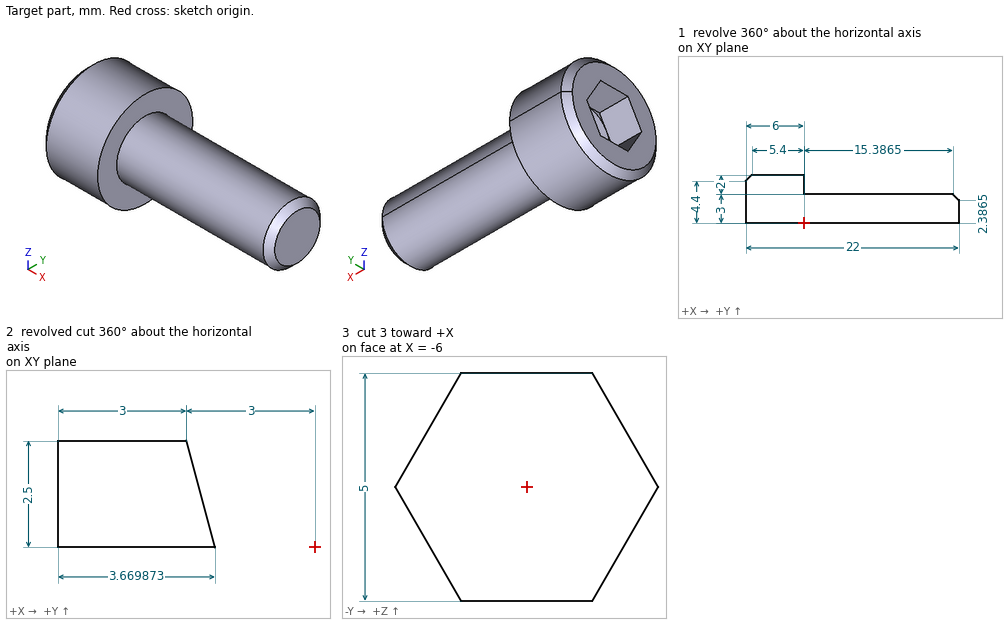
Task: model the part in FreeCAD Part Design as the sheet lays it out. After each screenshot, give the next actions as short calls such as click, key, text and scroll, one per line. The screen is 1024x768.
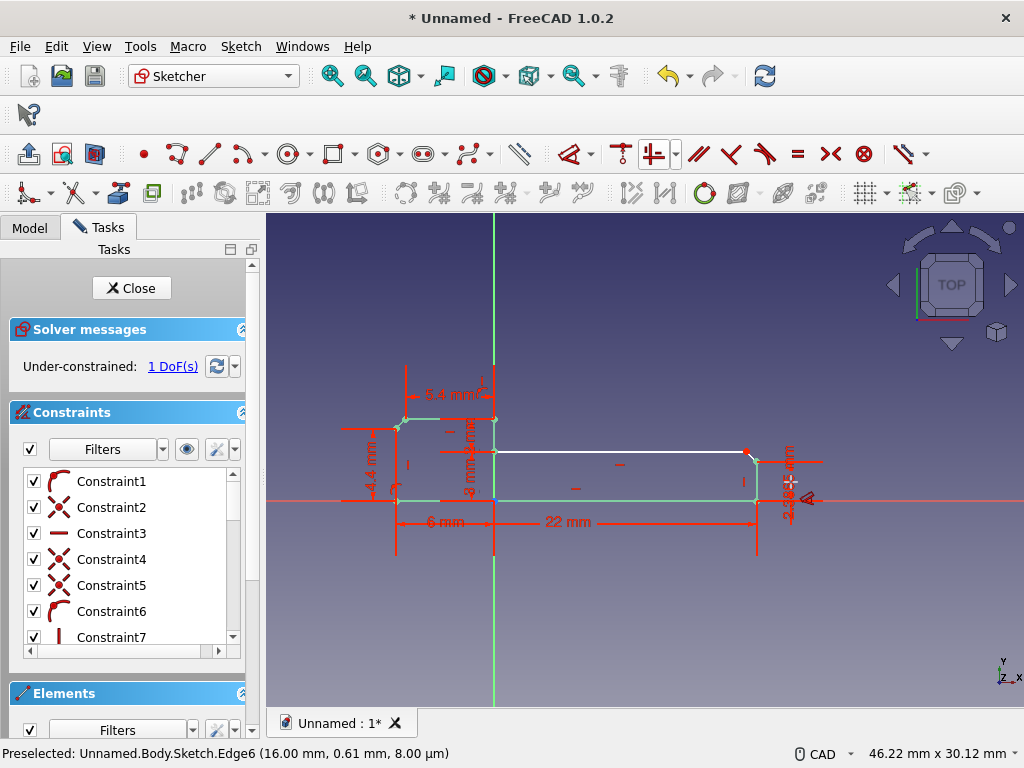
click(671, 452)
click(621, 418)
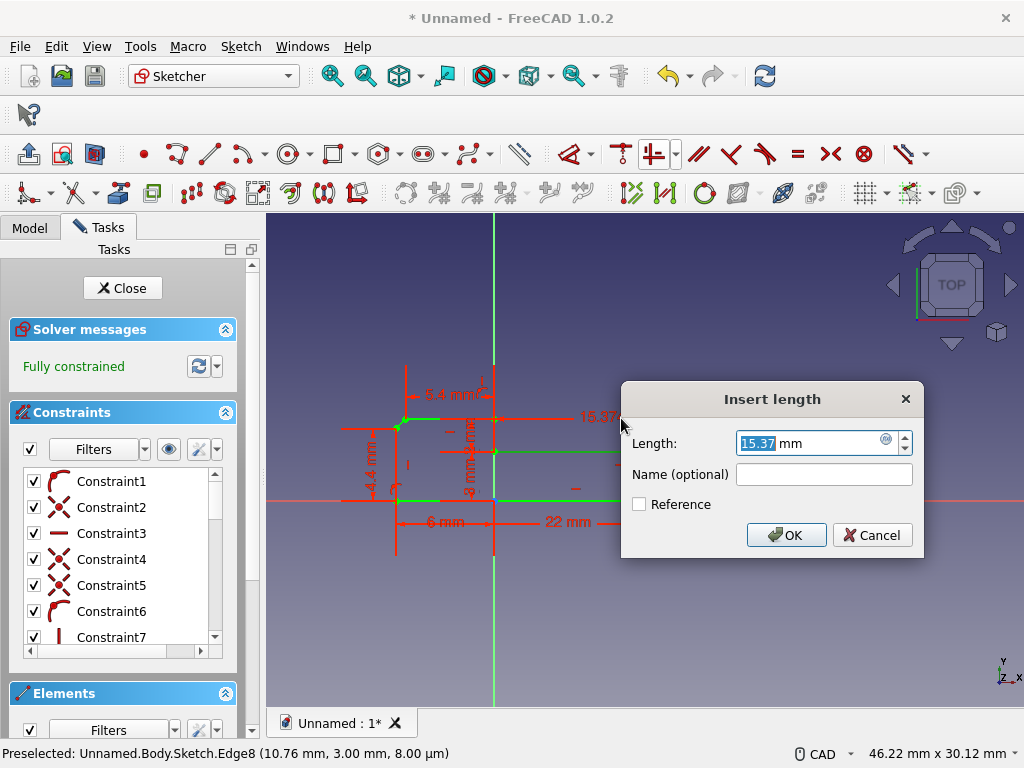
text(15.3865)
key(Return)
key(Escape)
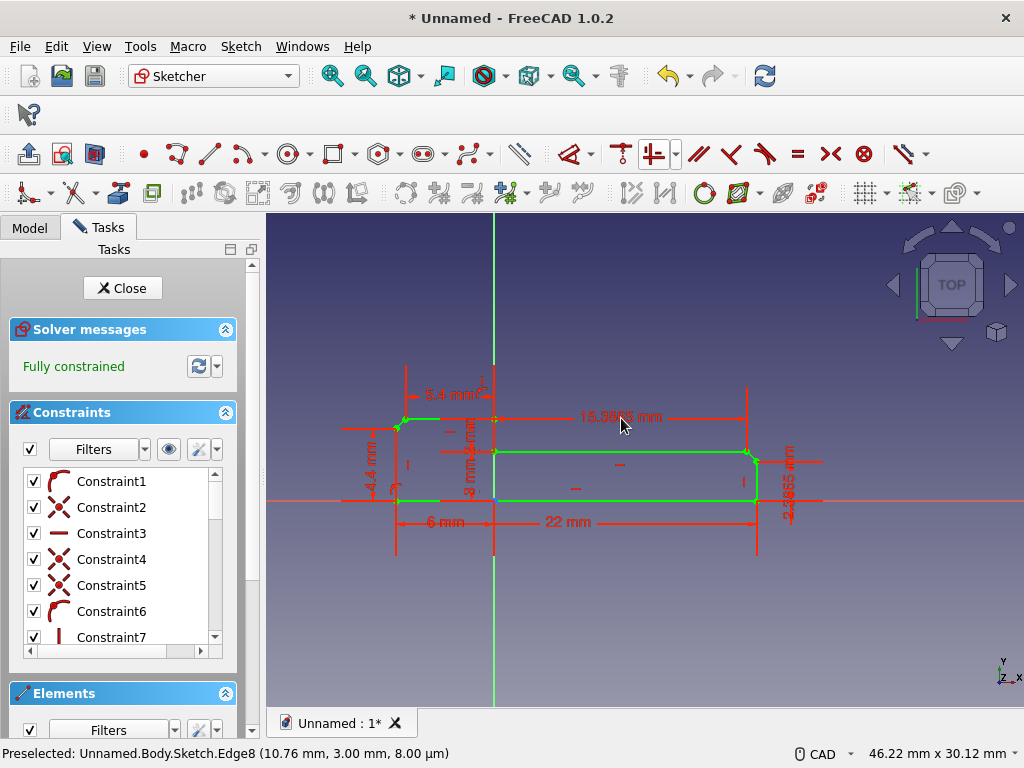
click(123, 288)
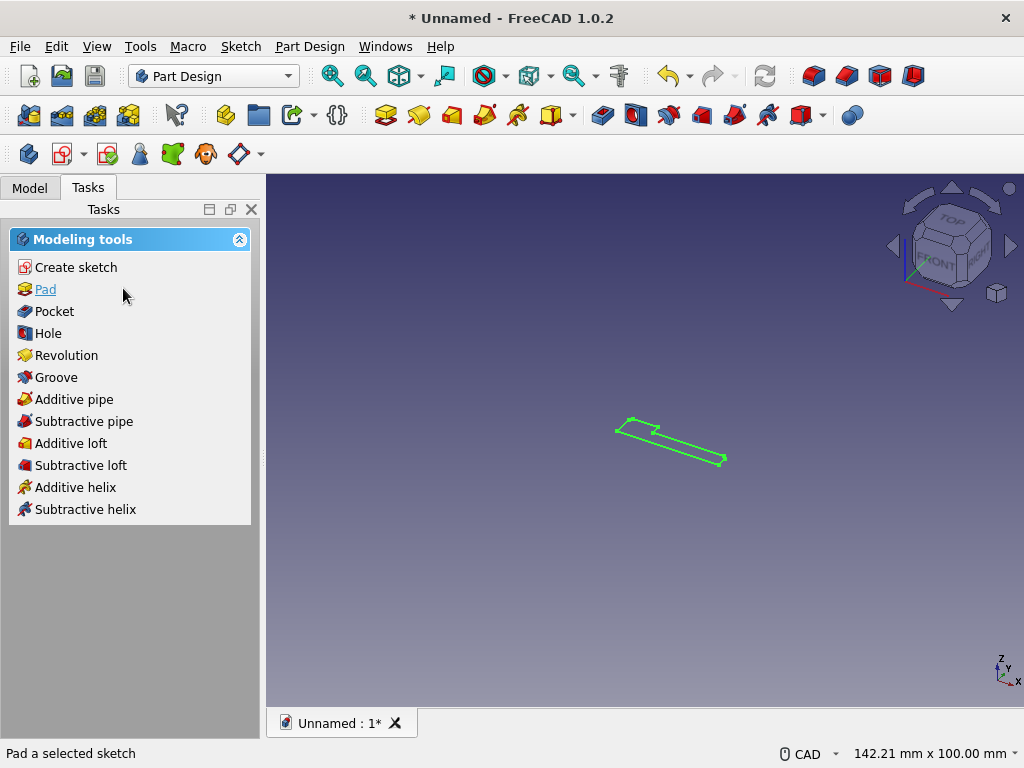
click(419, 116)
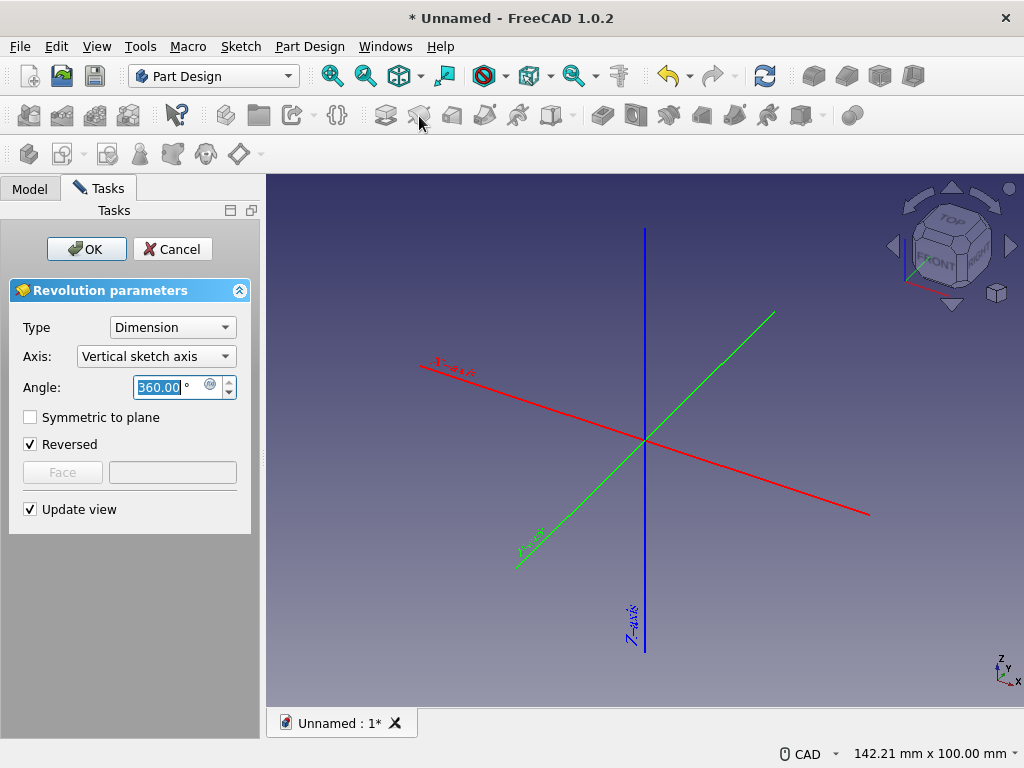
click(157, 356)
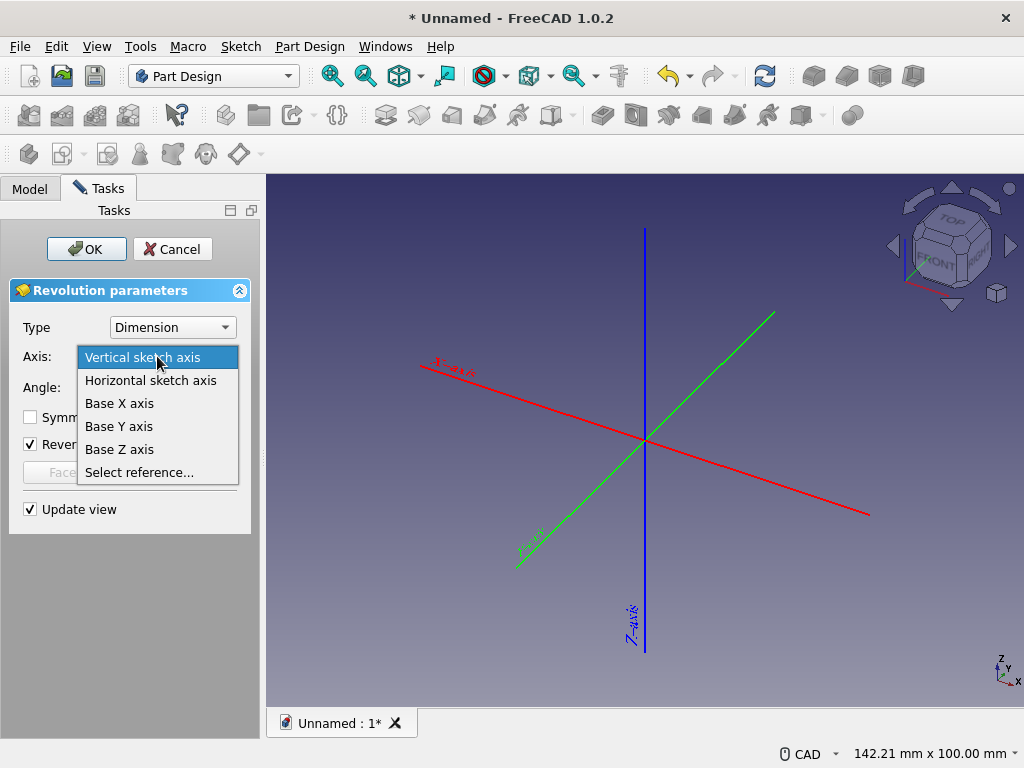
click(156, 380)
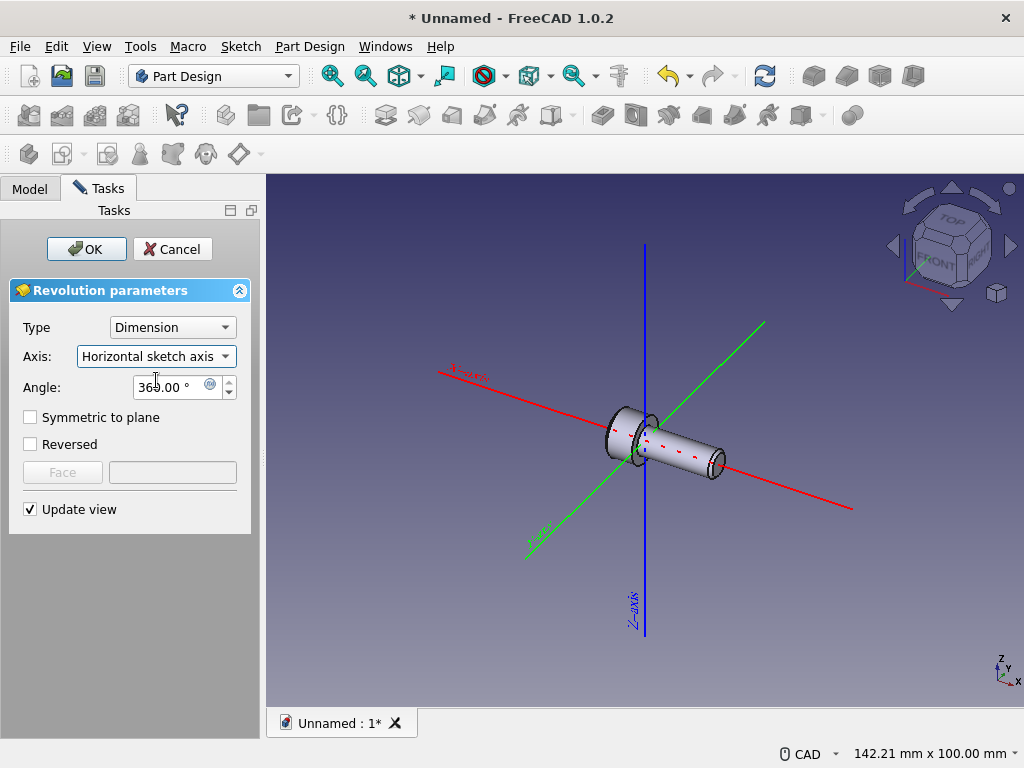
click(87, 249)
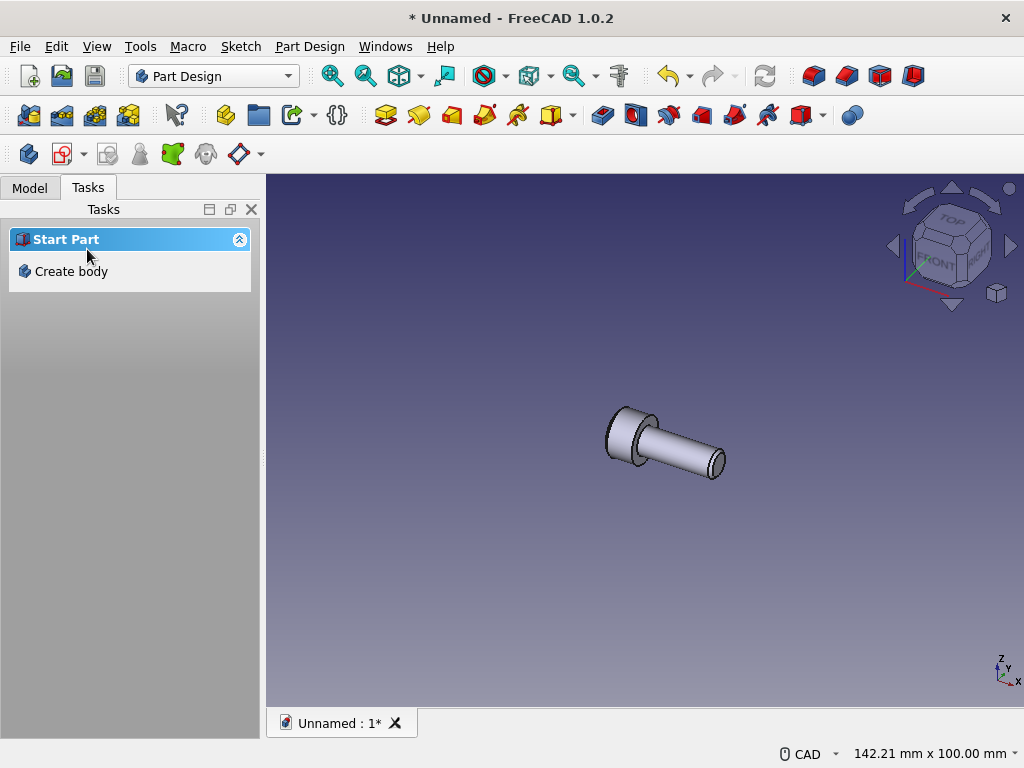
click(333, 76)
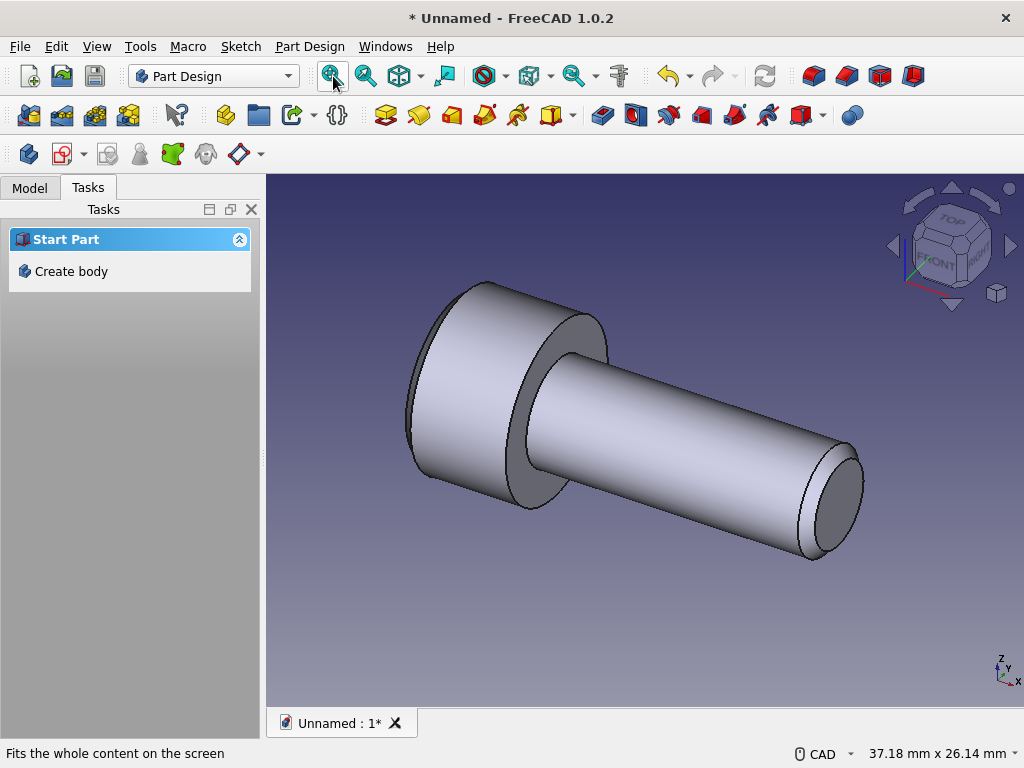
click(62, 154)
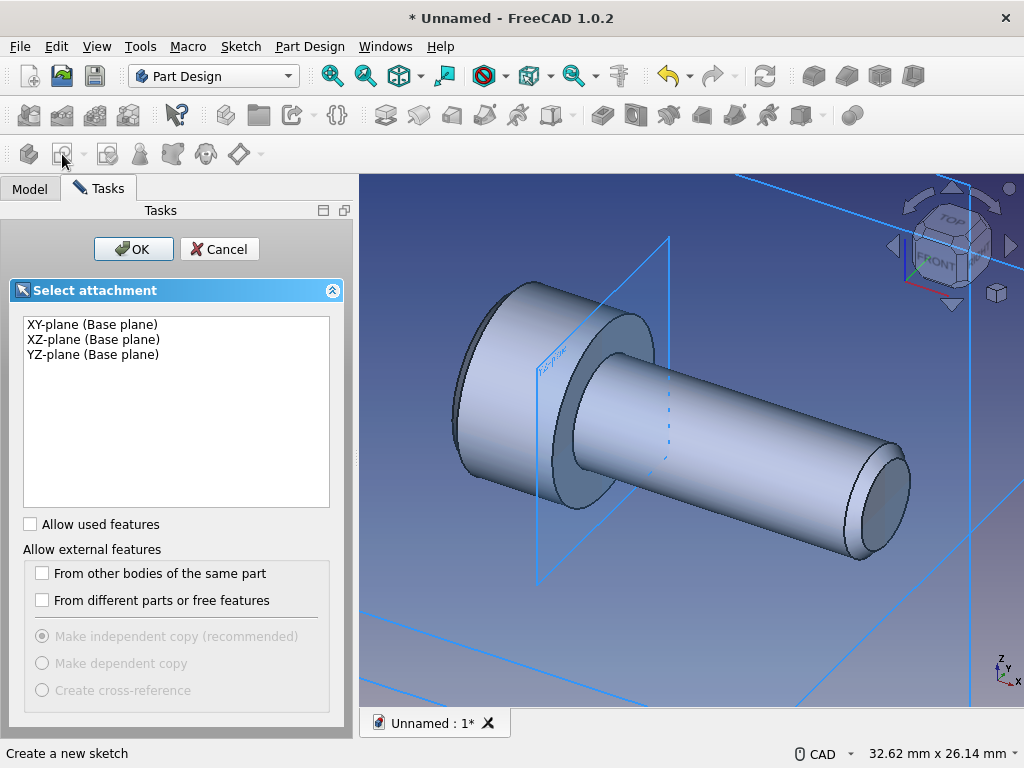
click(84, 324)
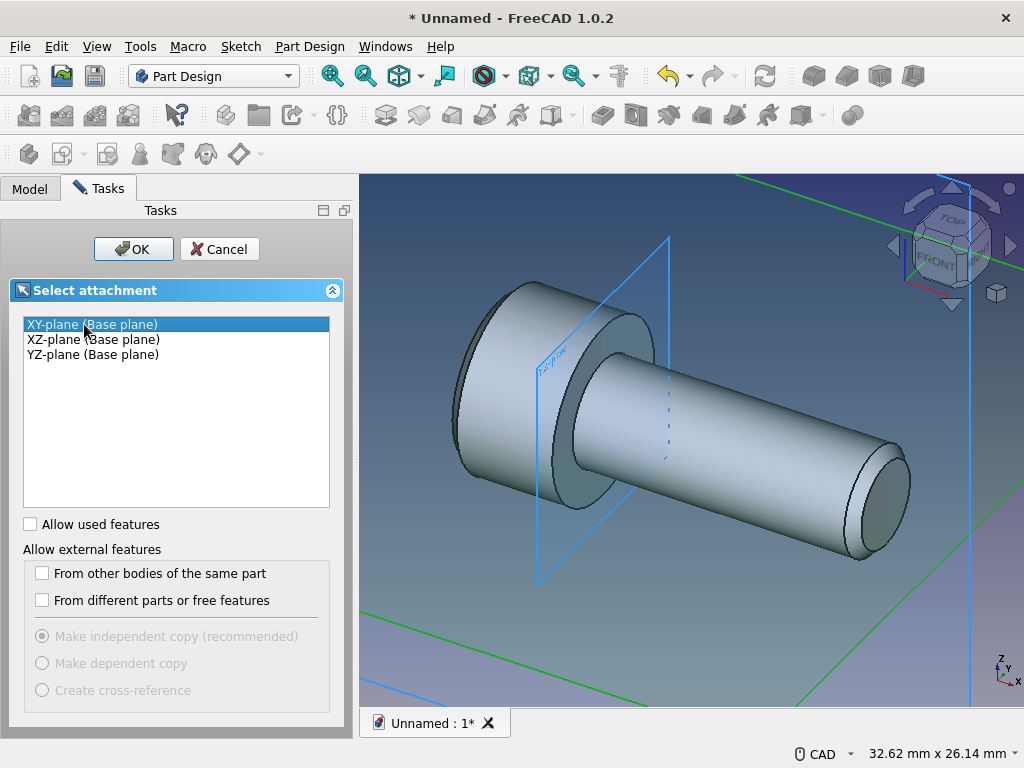
click(134, 249)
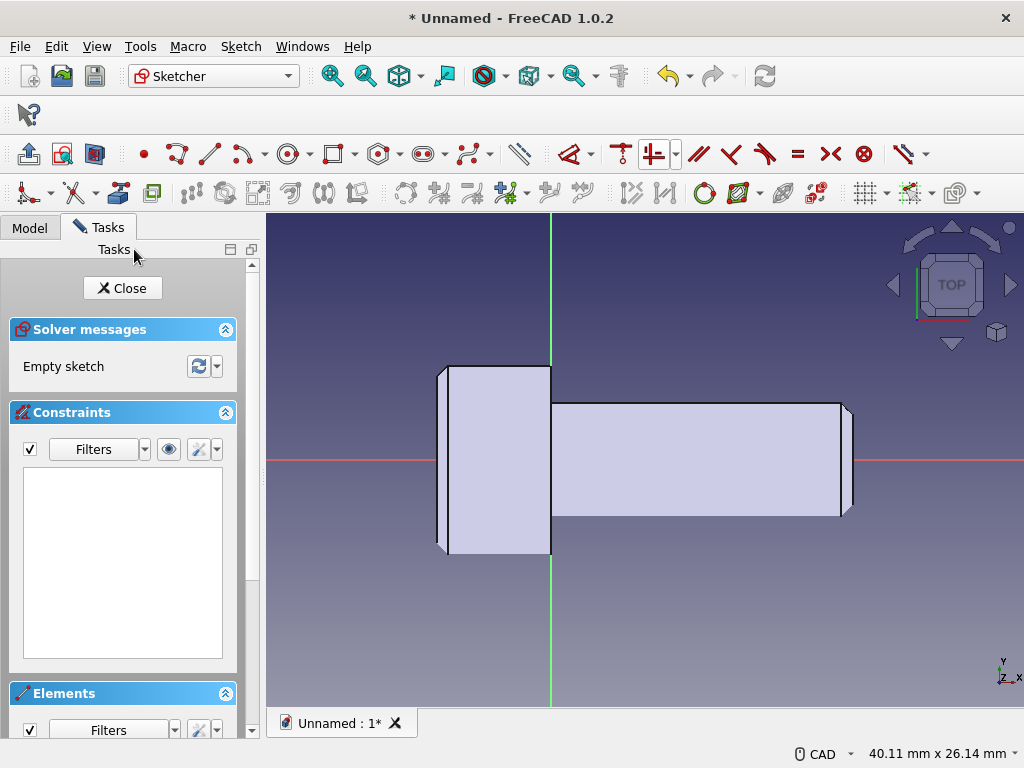
click(95, 154)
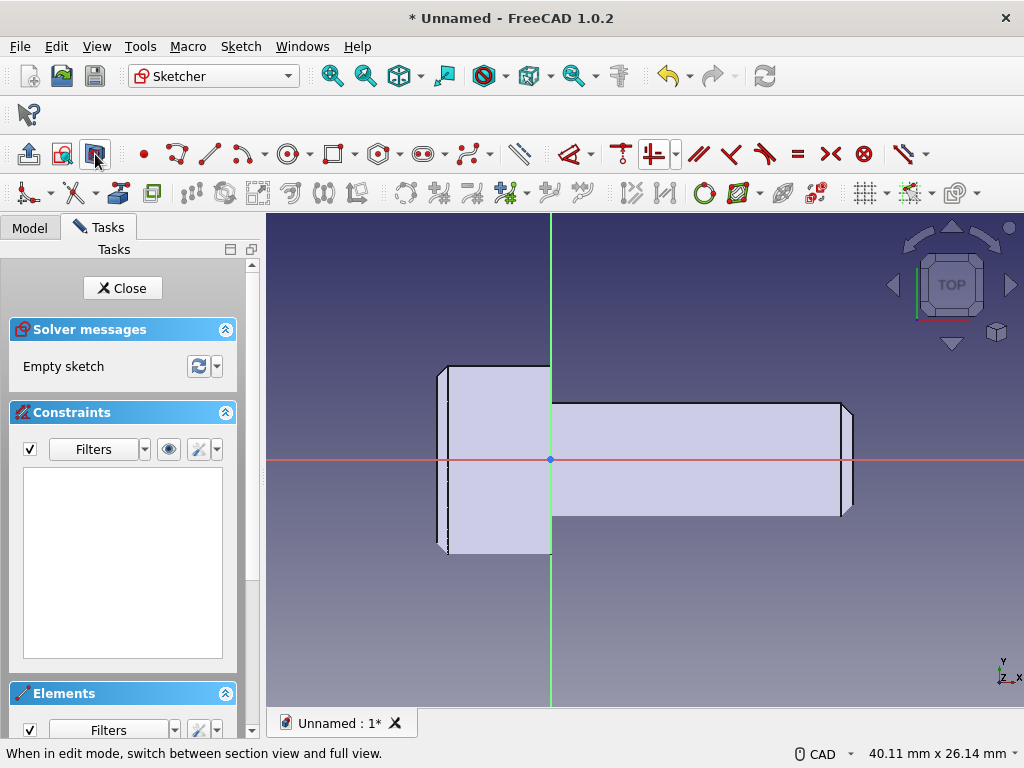
scroll(458, 426, up, 6)